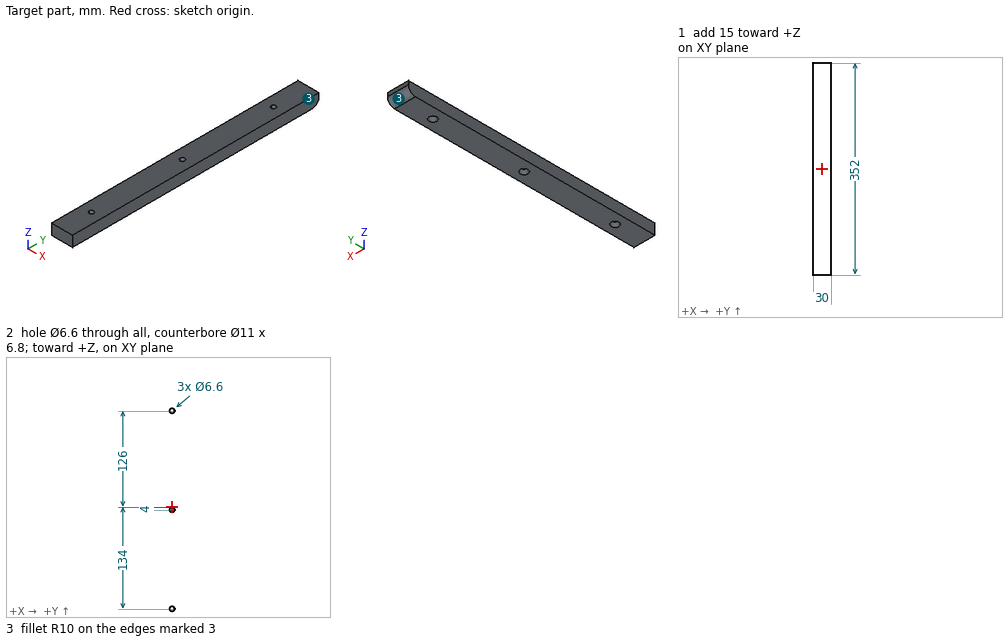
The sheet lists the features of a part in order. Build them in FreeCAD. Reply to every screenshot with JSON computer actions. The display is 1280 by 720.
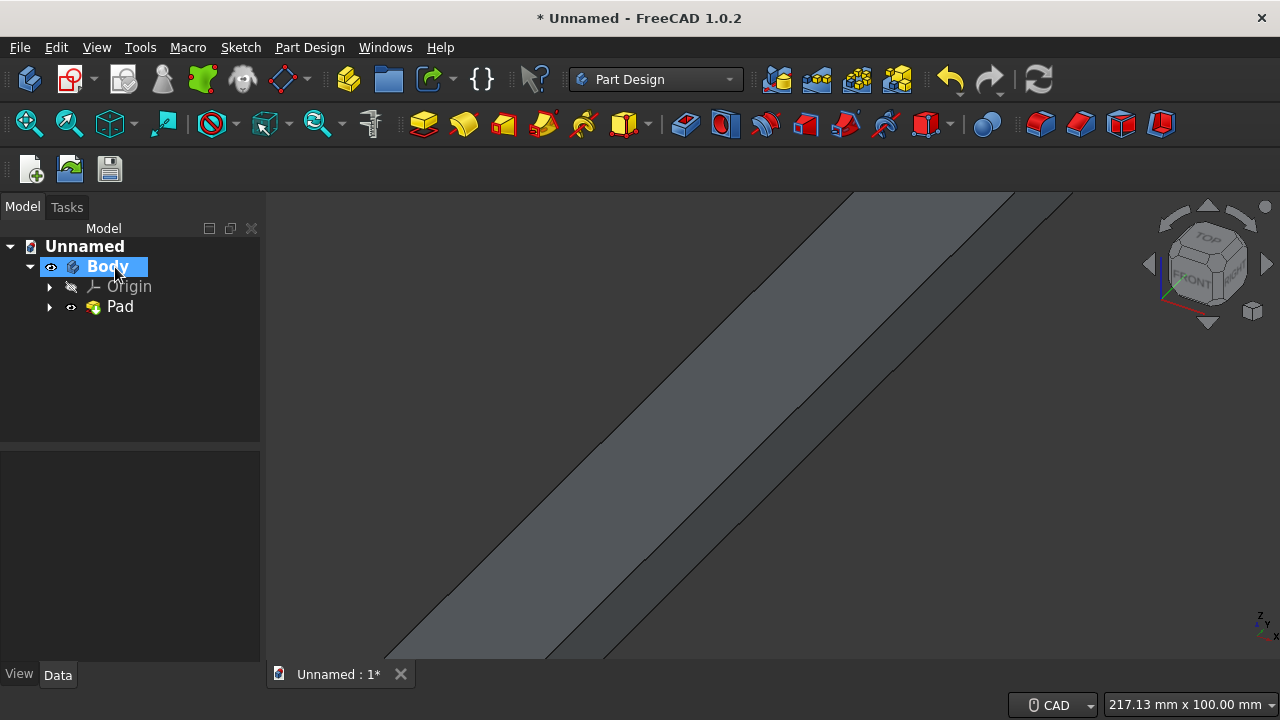
{"action": "key", "text": "v f"}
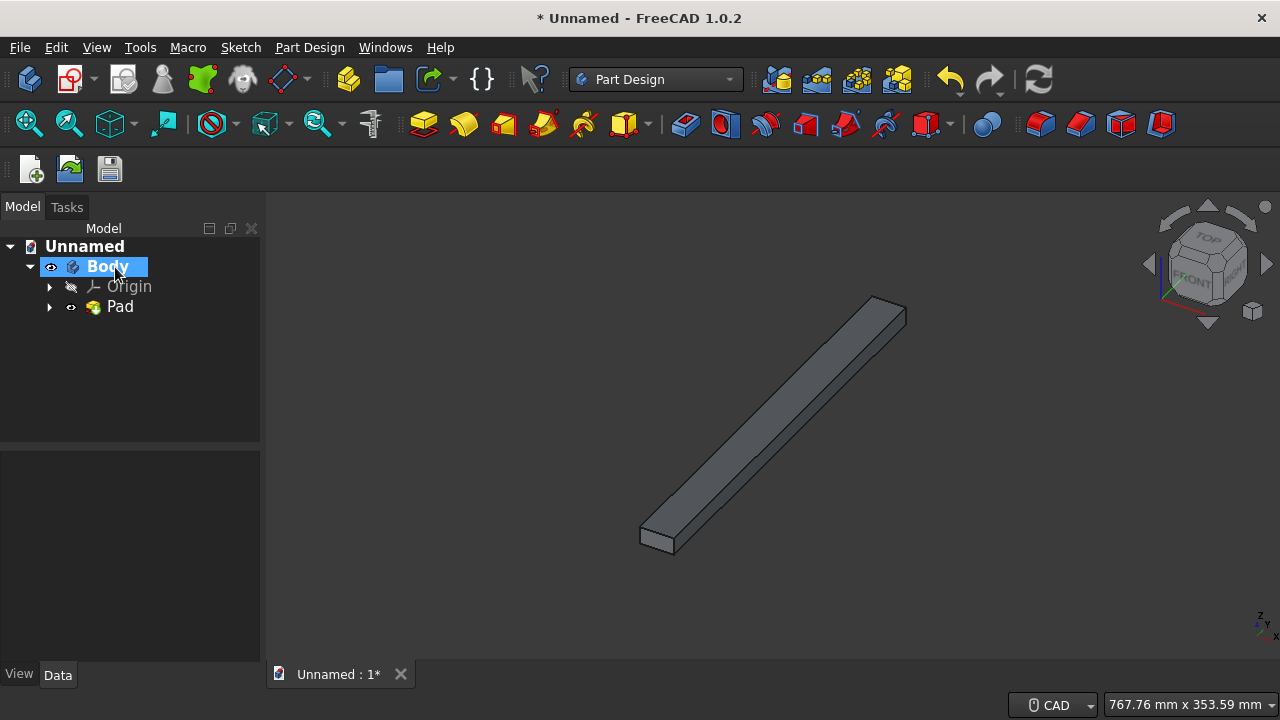
{"action": "left_click", "coordinate": [70, 80]}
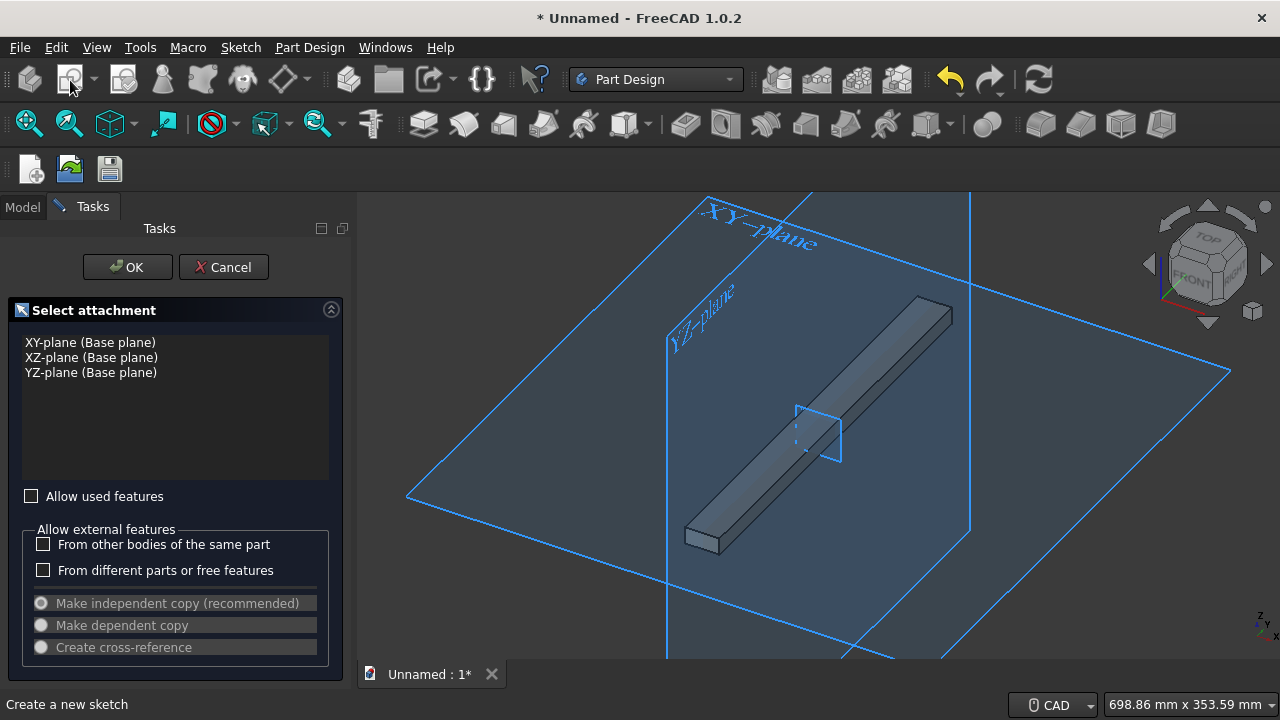
{"action": "left_click", "coordinate": [82, 342]}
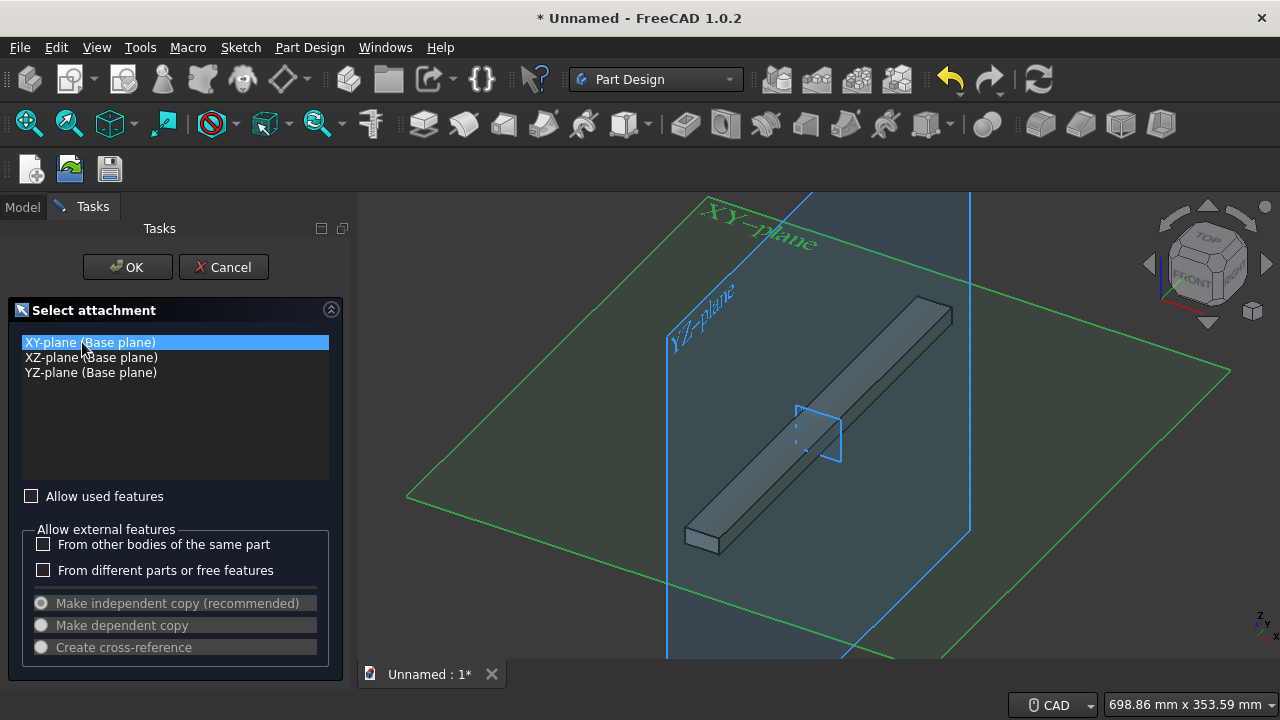
{"action": "left_click", "coordinate": [128, 267]}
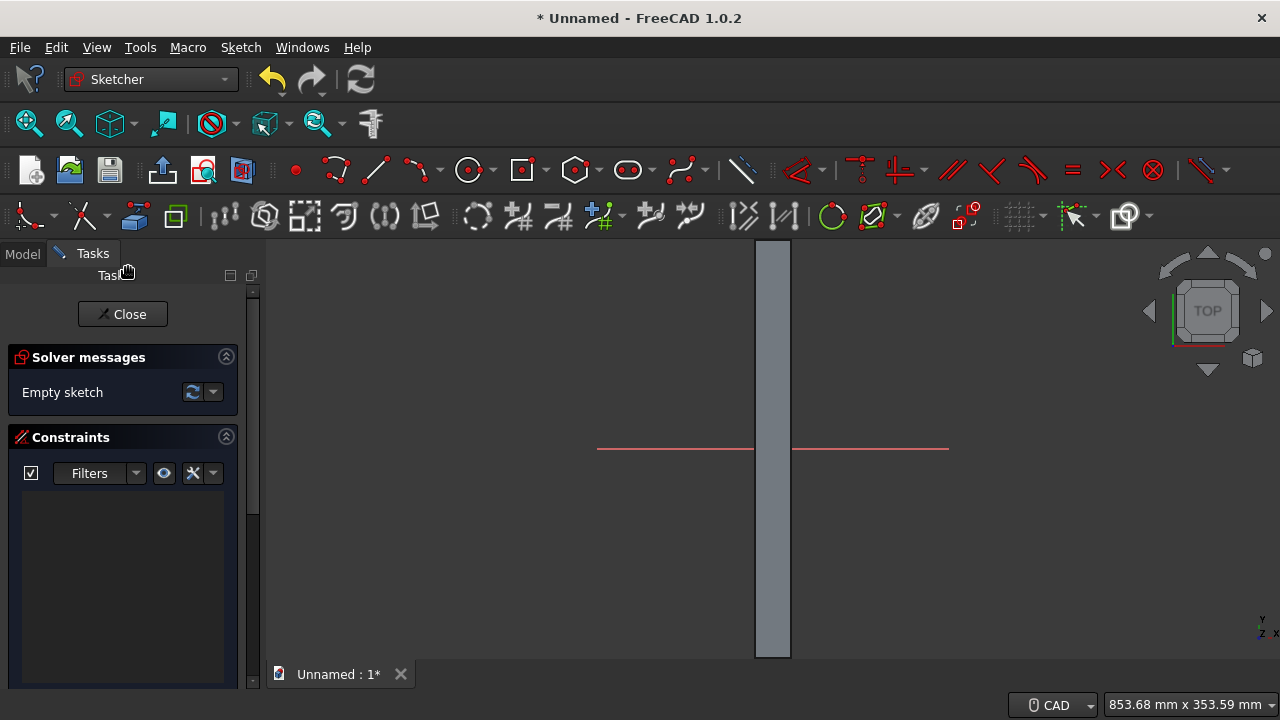
{"action": "left_click", "coordinate": [244, 170]}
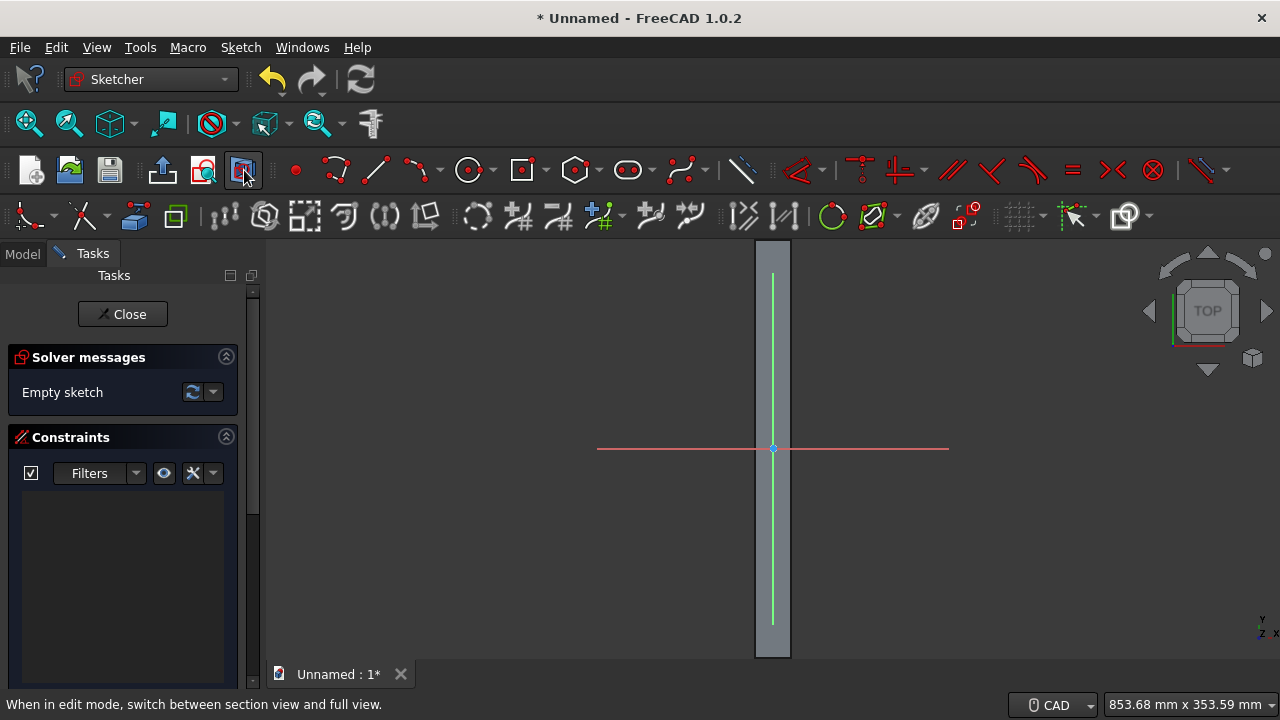
{"action": "scroll", "coordinate": [395, 428], "scroll_direction": "down", "scroll_amount": 1}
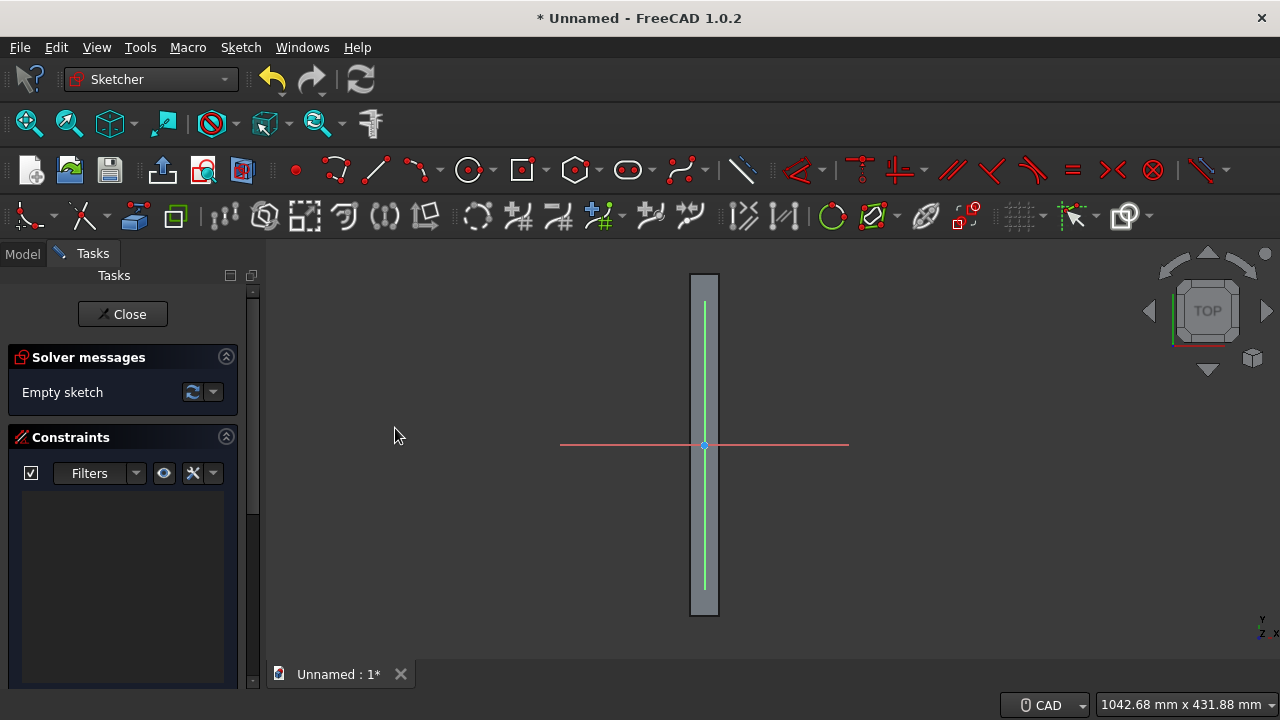
{"action": "left_click", "coordinate": [470, 170]}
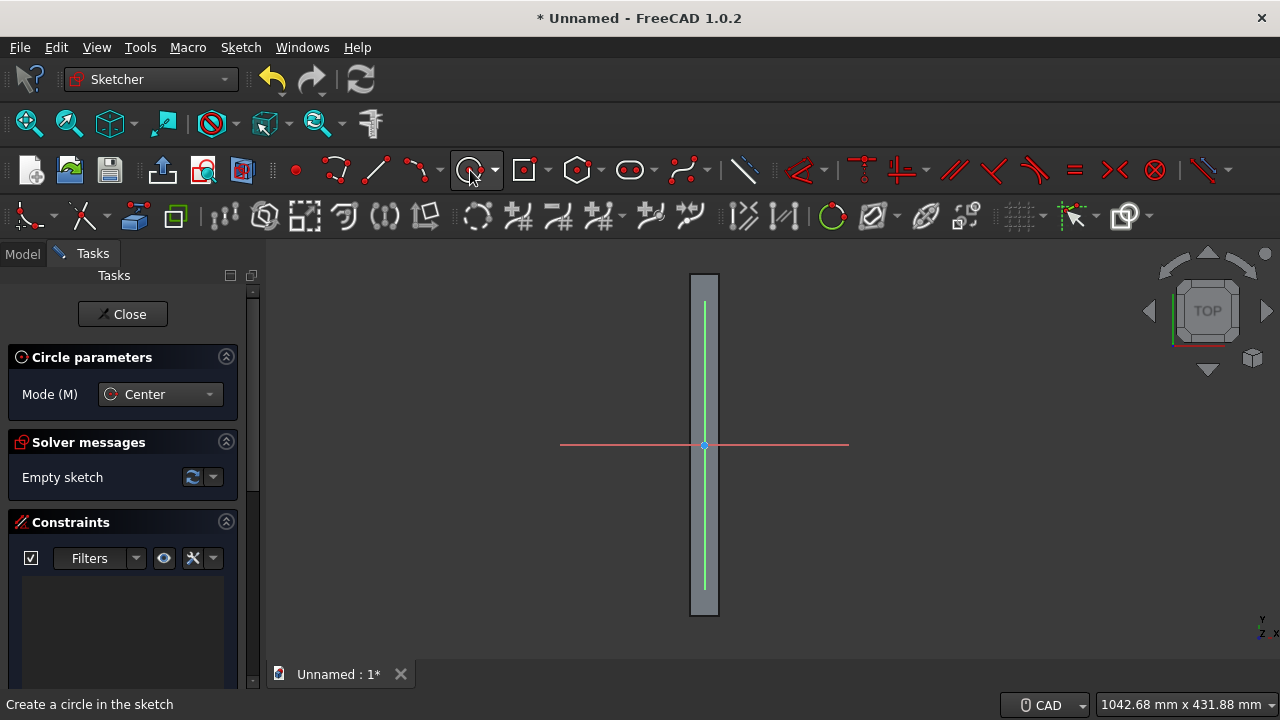
{"action": "scroll", "coordinate": [705, 323], "scroll_direction": "up", "scroll_amount": 10}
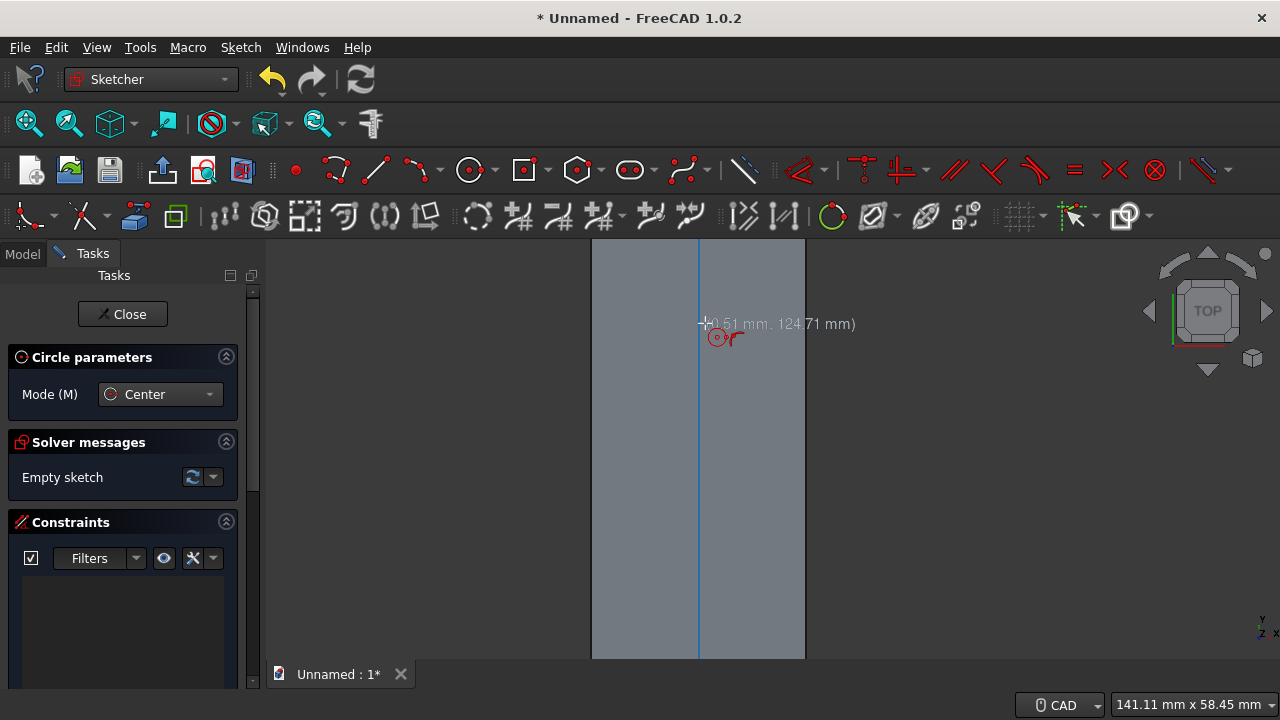
{"action": "scroll", "coordinate": [705, 323], "scroll_direction": "down", "scroll_amount": 10}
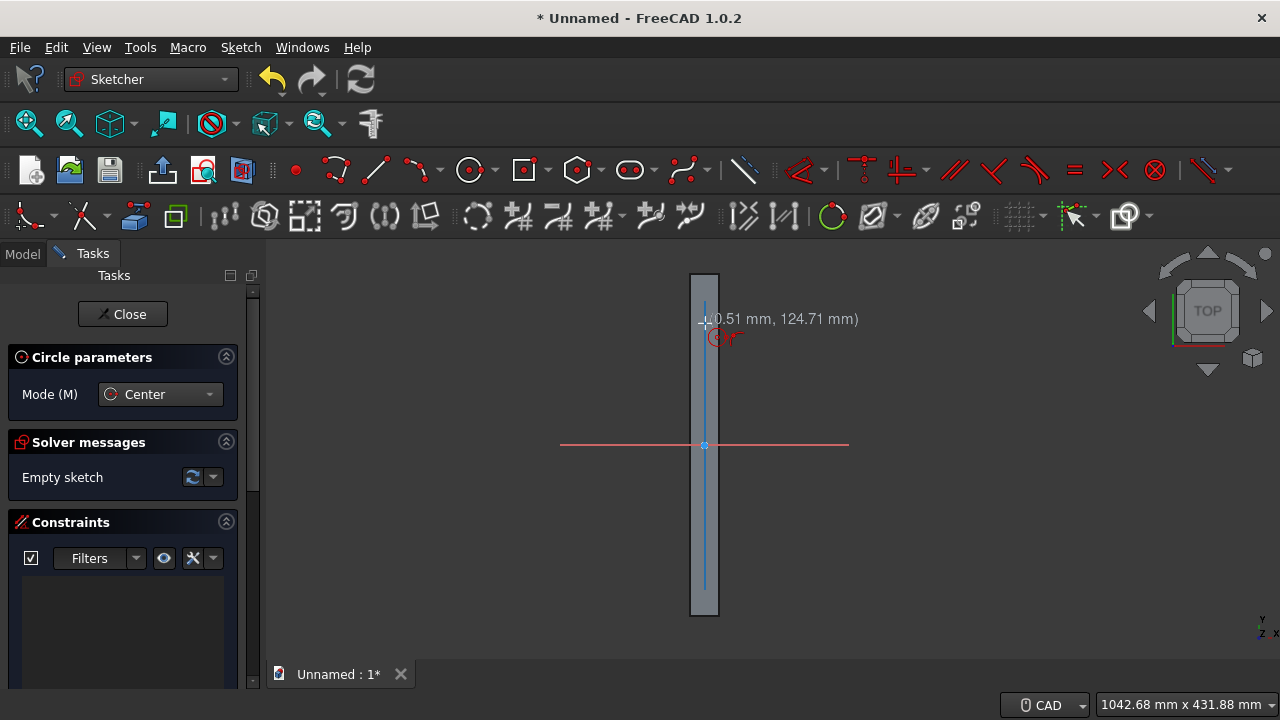
{"action": "left_click", "coordinate": [705, 323]}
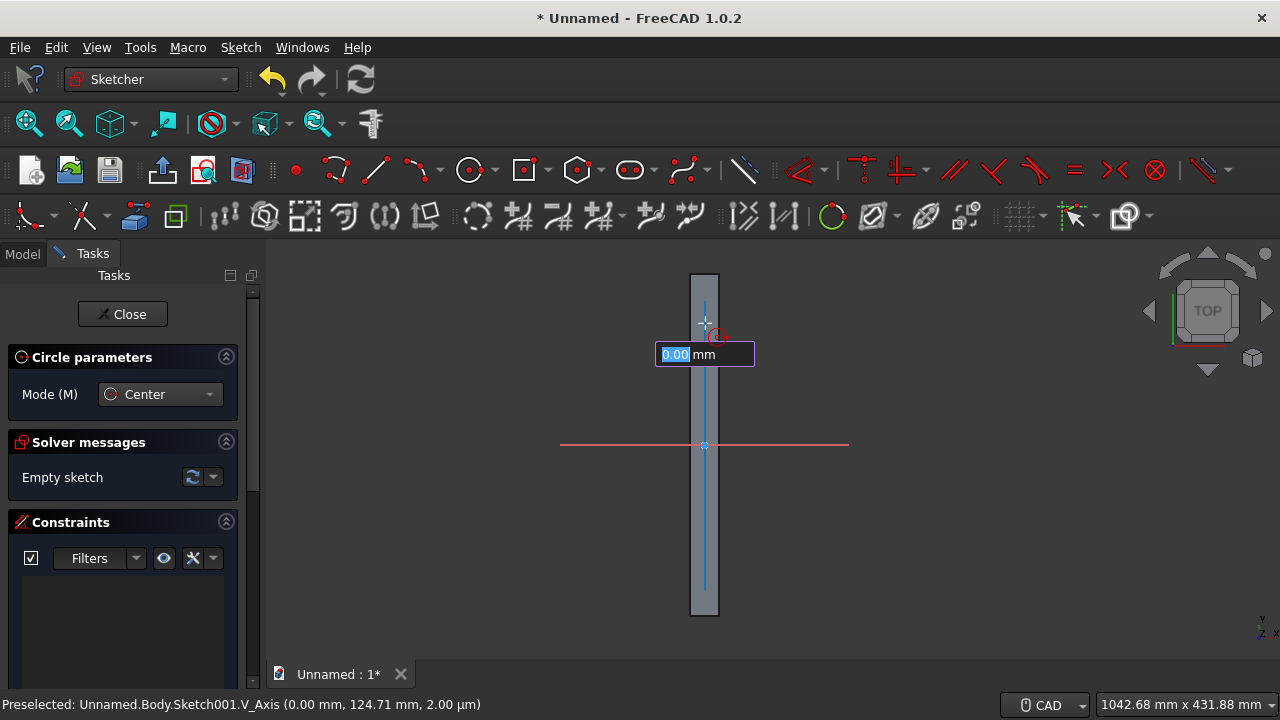
{"action": "scroll", "coordinate": [708, 322], "scroll_direction": "up", "scroll_amount": 9}
{"action": "mouse_move", "coordinate": [703, 319]}